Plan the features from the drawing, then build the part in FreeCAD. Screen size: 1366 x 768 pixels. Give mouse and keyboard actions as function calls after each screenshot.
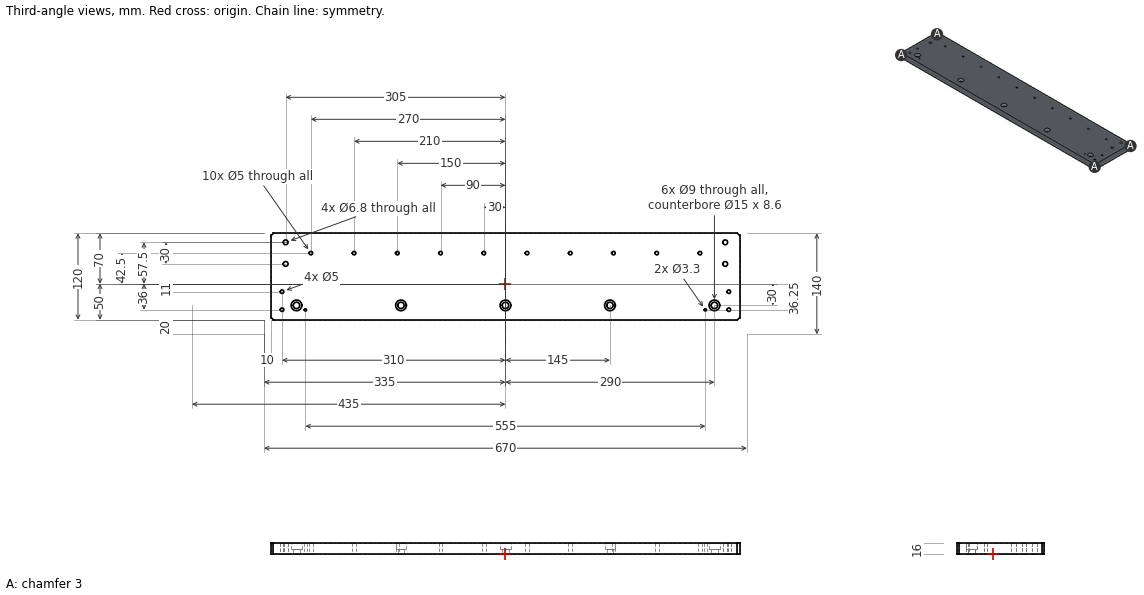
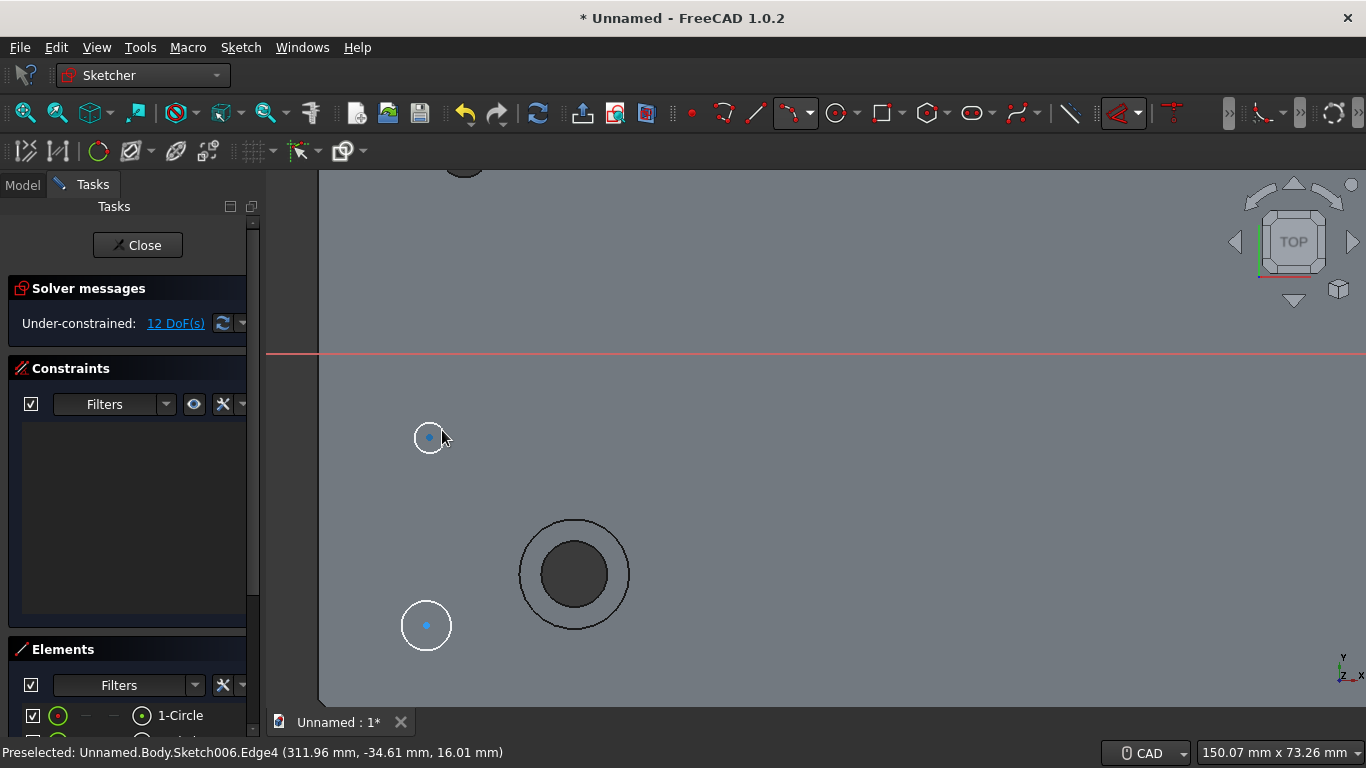
click(440, 427)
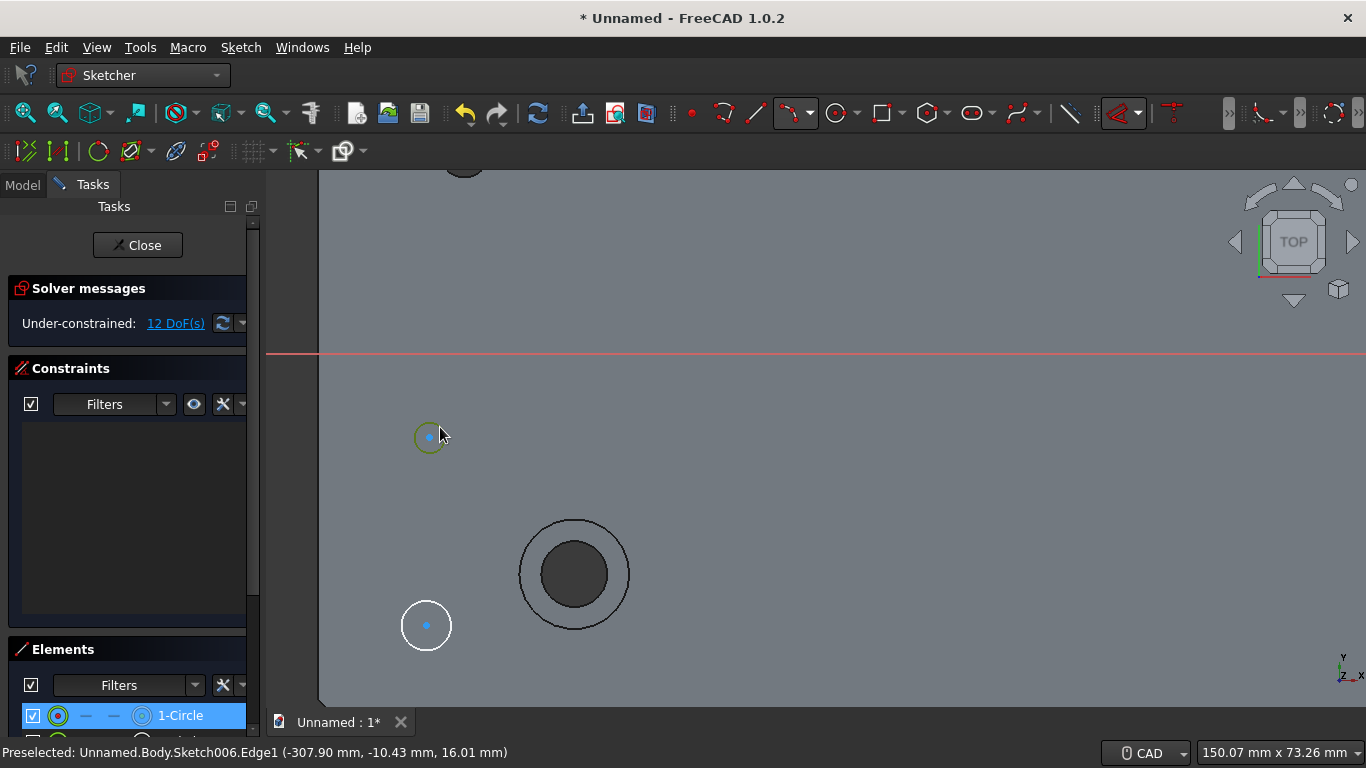
click(444, 608)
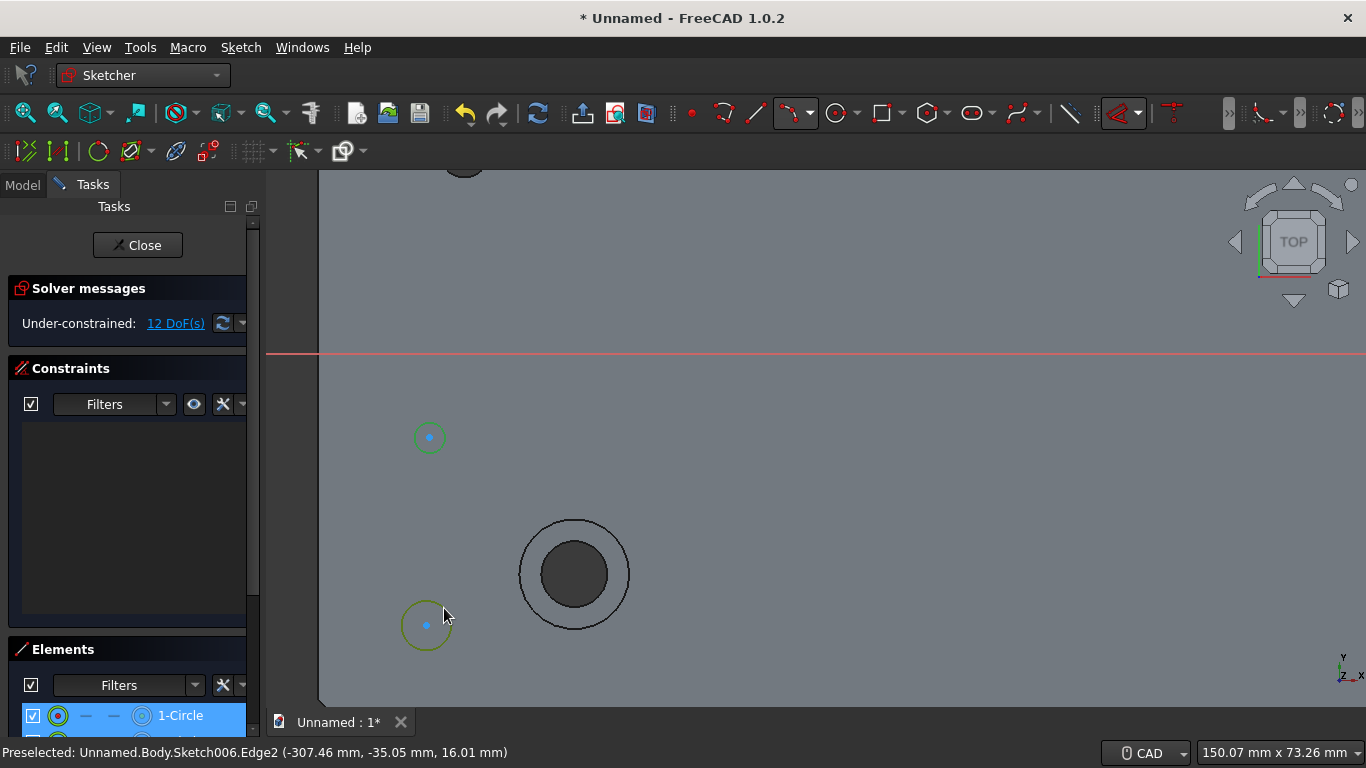
scroll(442, 430, down, 10)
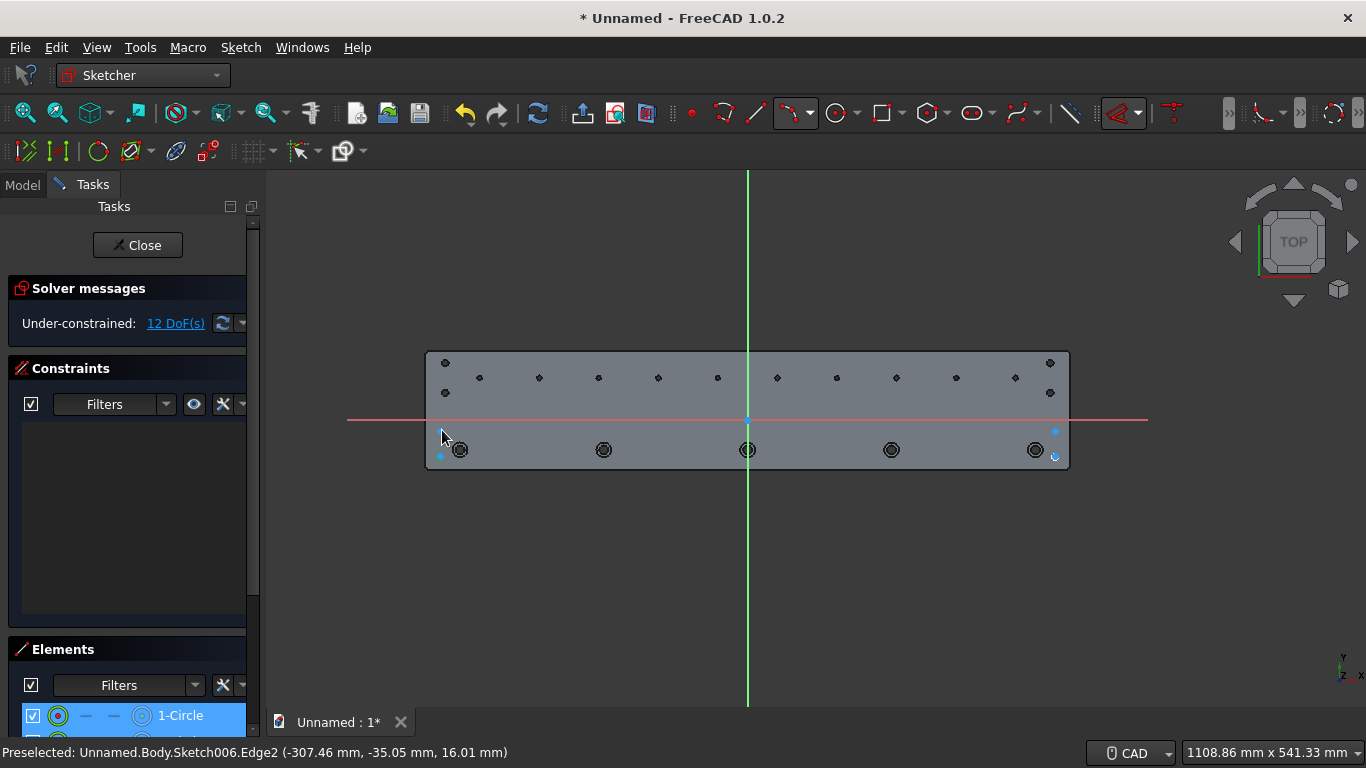
scroll(1057, 430, up, 10)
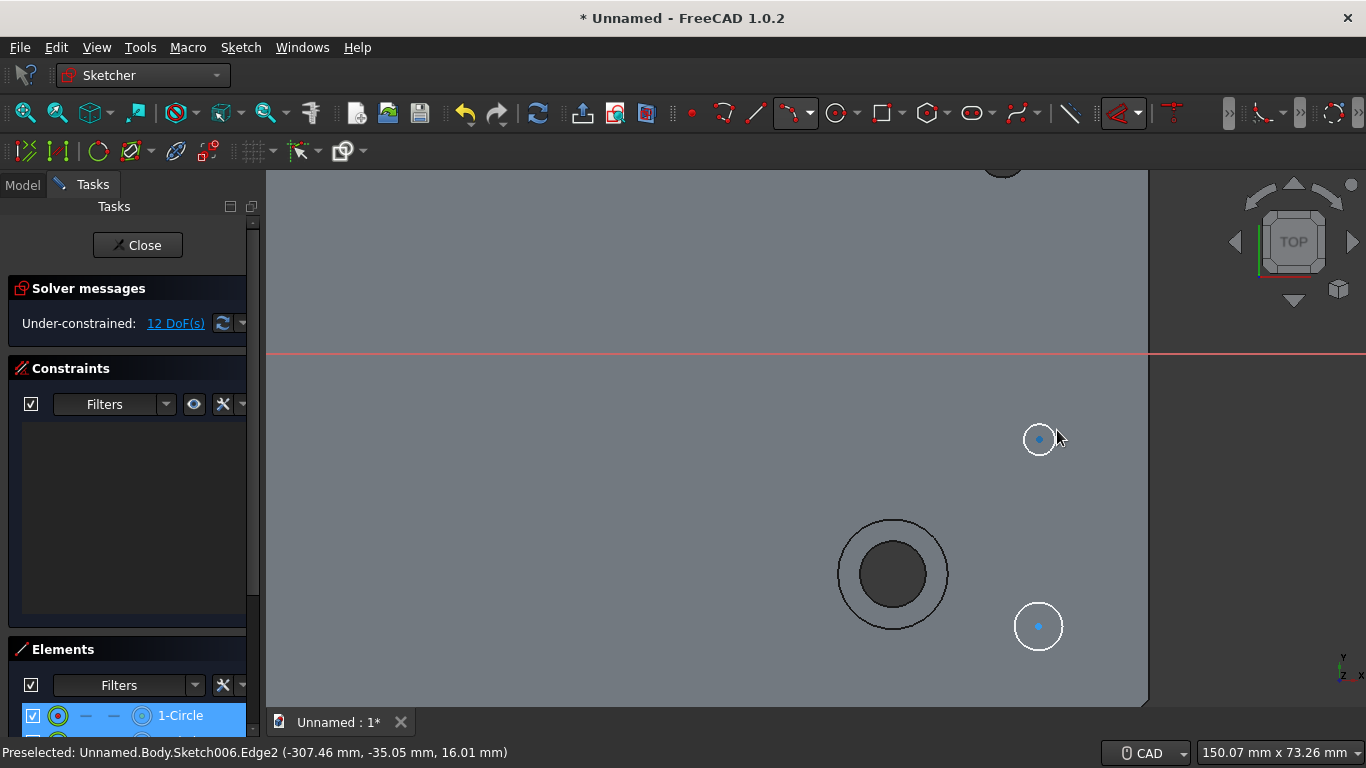
click(1050, 429)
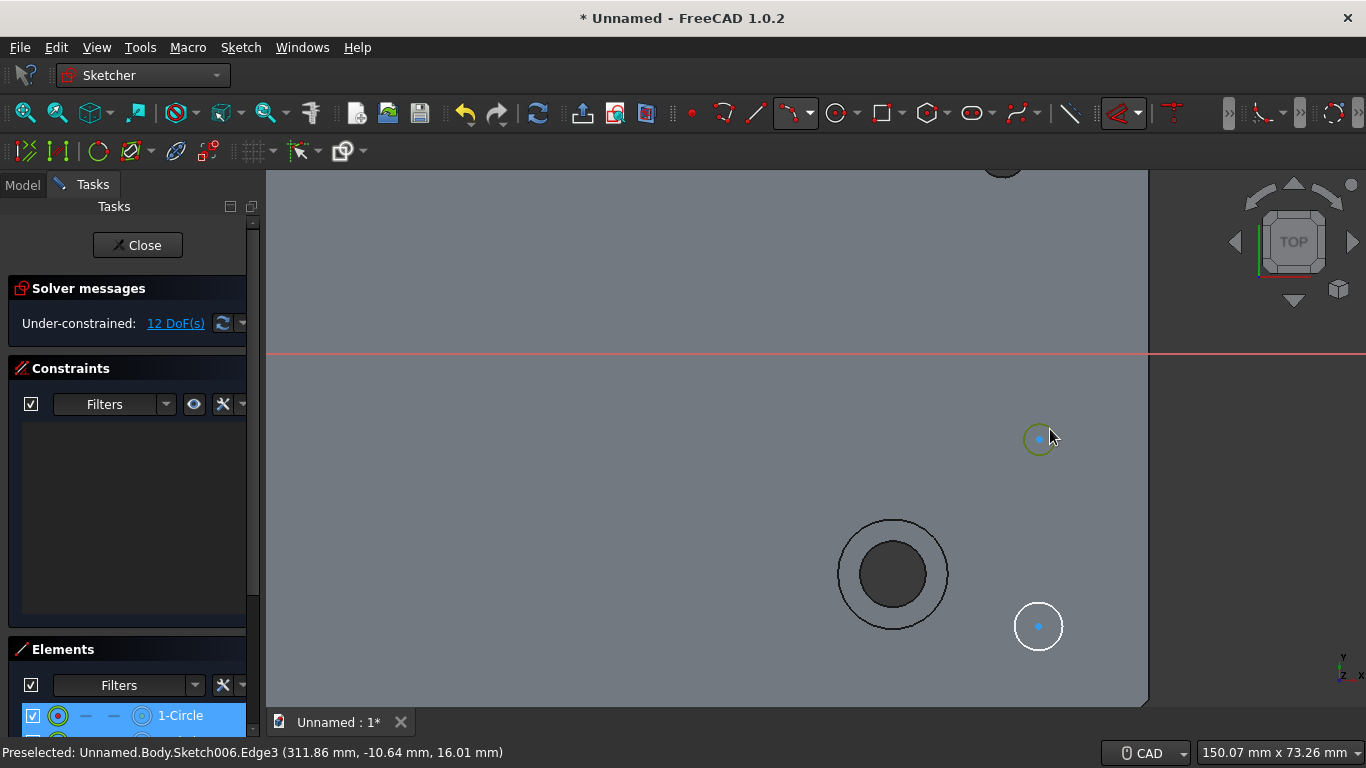
click(1055, 609)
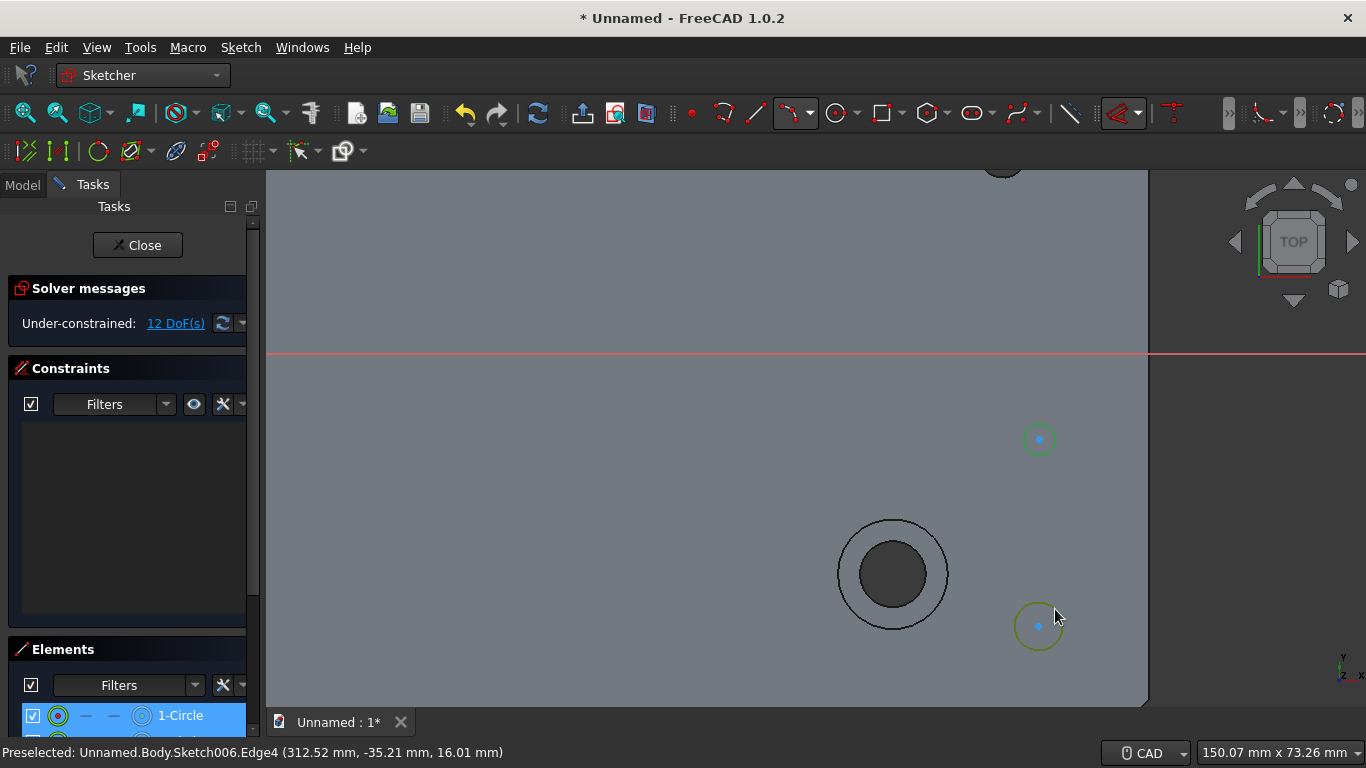
key(e)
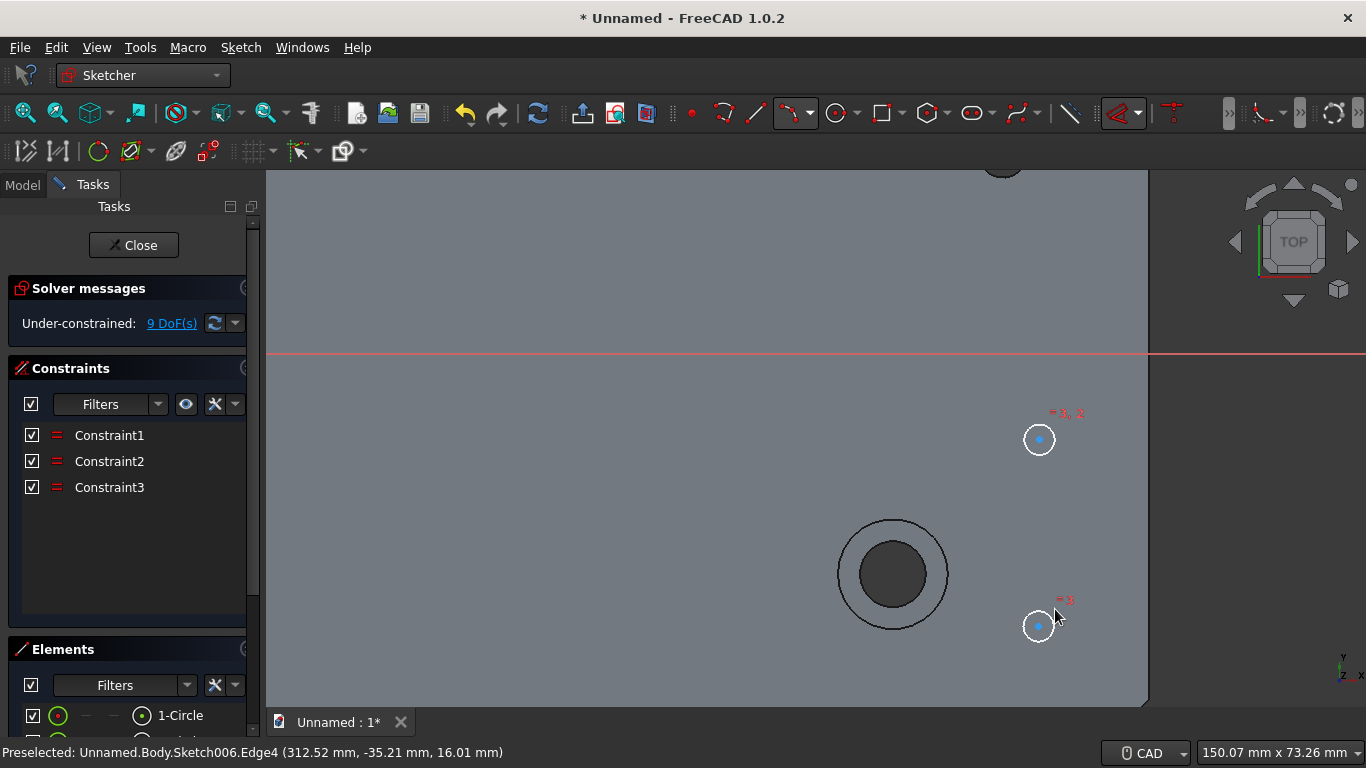
scroll(1057, 430, down, 10)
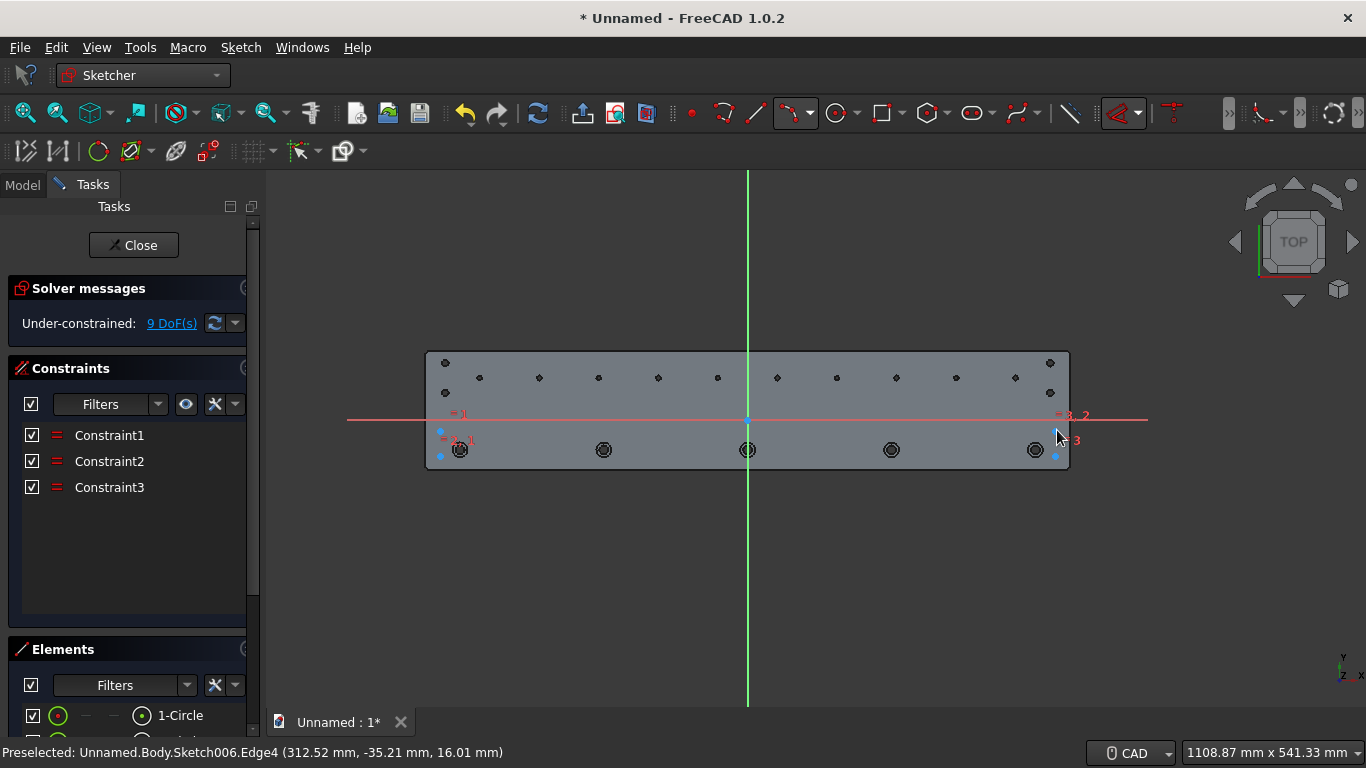
click(440, 432)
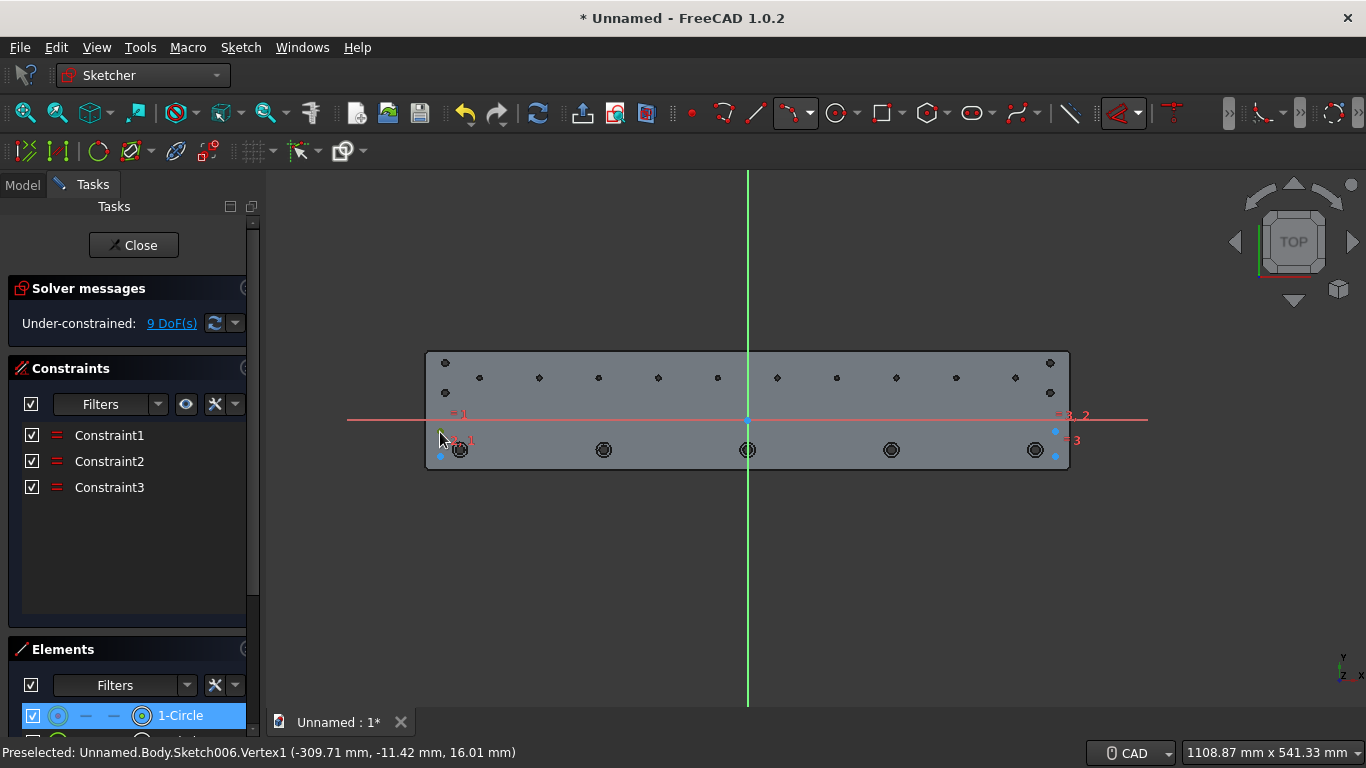
click(1055, 432)